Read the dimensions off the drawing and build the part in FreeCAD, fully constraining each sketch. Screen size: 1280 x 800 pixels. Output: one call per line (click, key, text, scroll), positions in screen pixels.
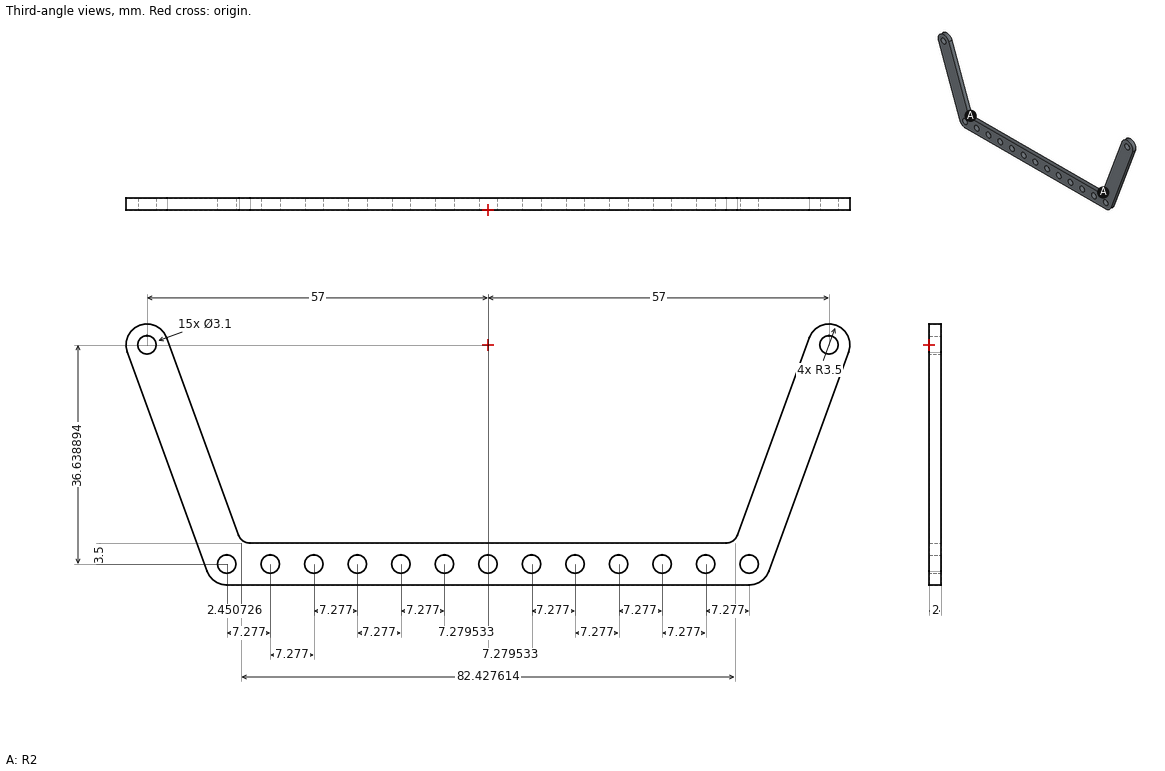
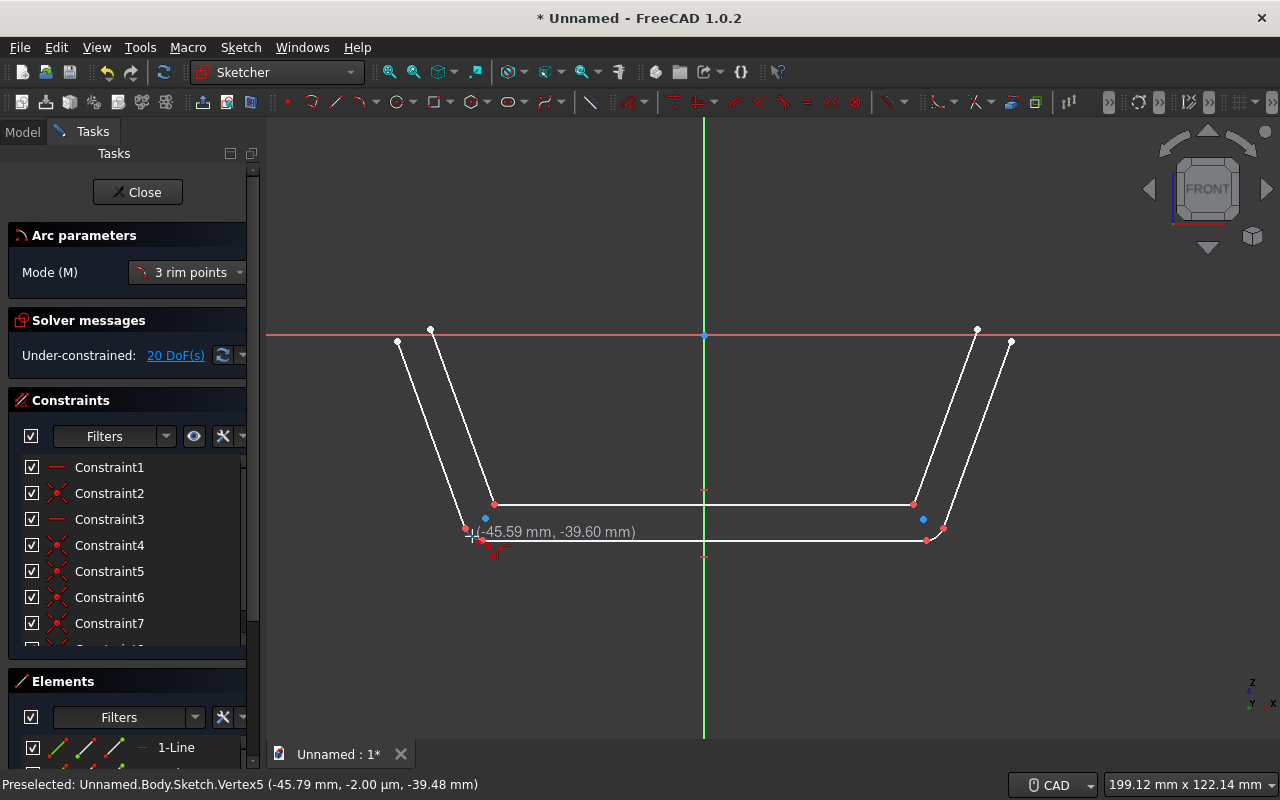
scroll(397, 341, up, 5)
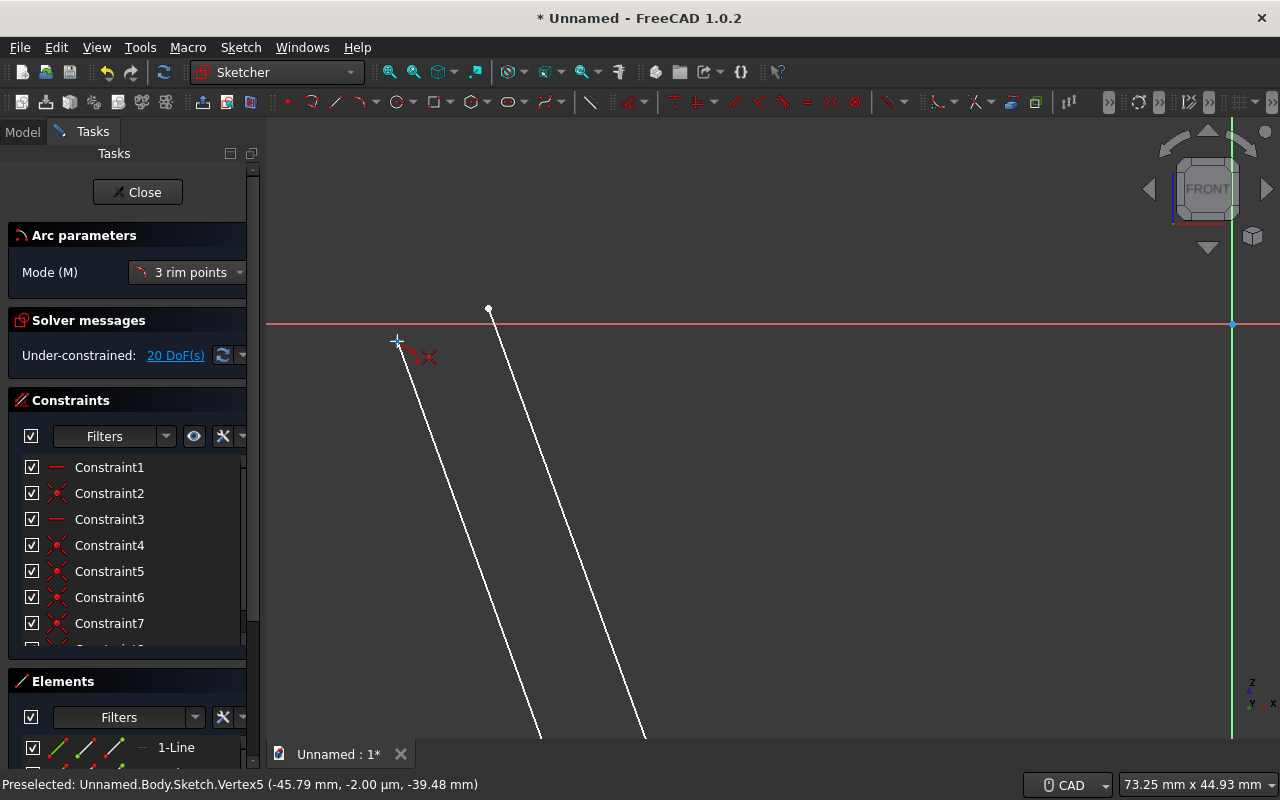
click(398, 341)
click(489, 308)
click(427, 279)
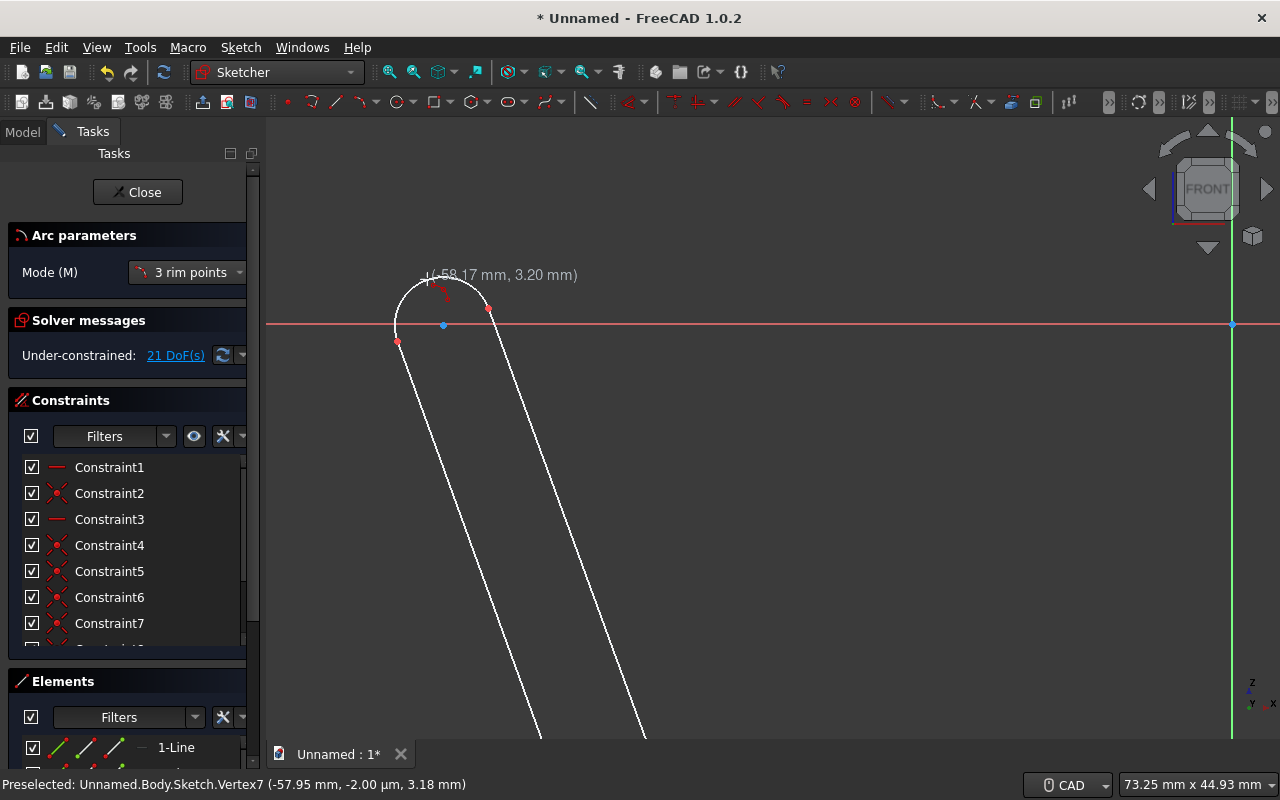
scroll(397, 340, down, 5)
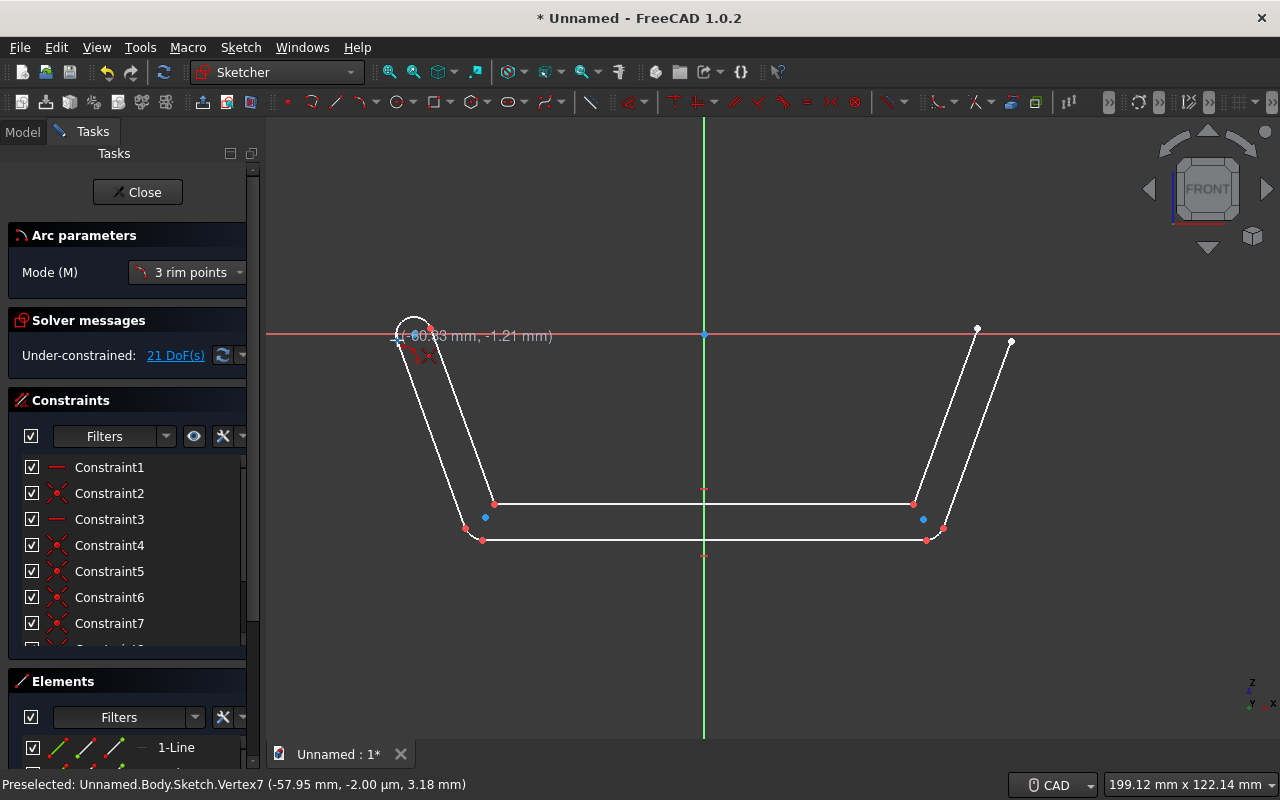
scroll(978, 328, up, 5)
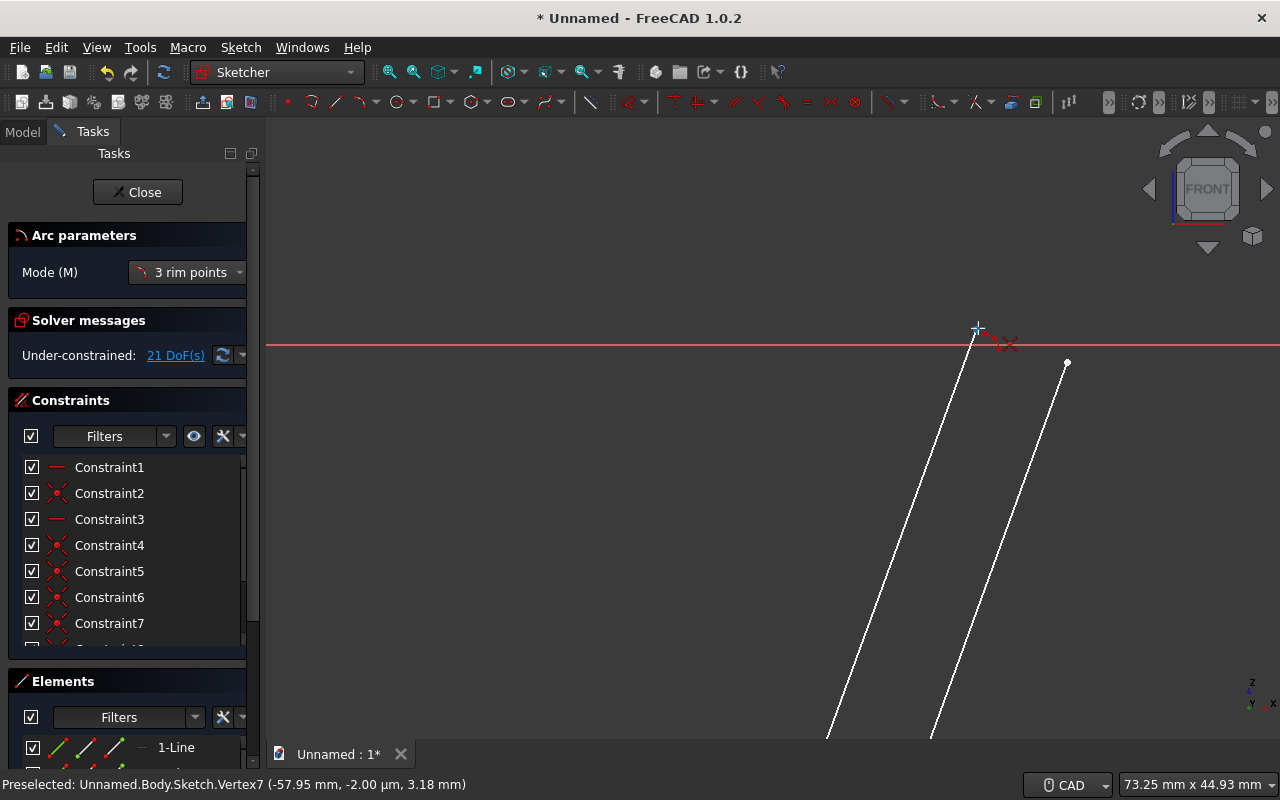
click(977, 329)
click(1067, 363)
click(1039, 299)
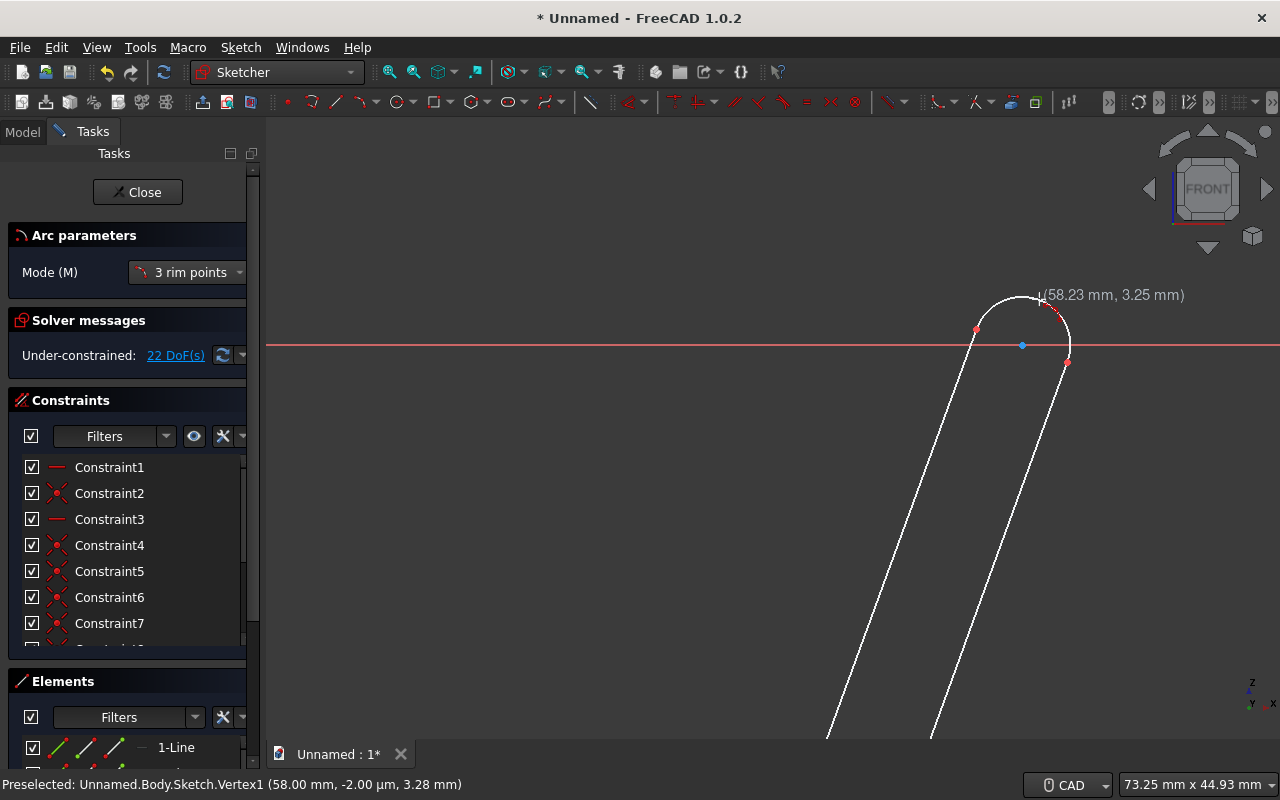
key(g)
key(c)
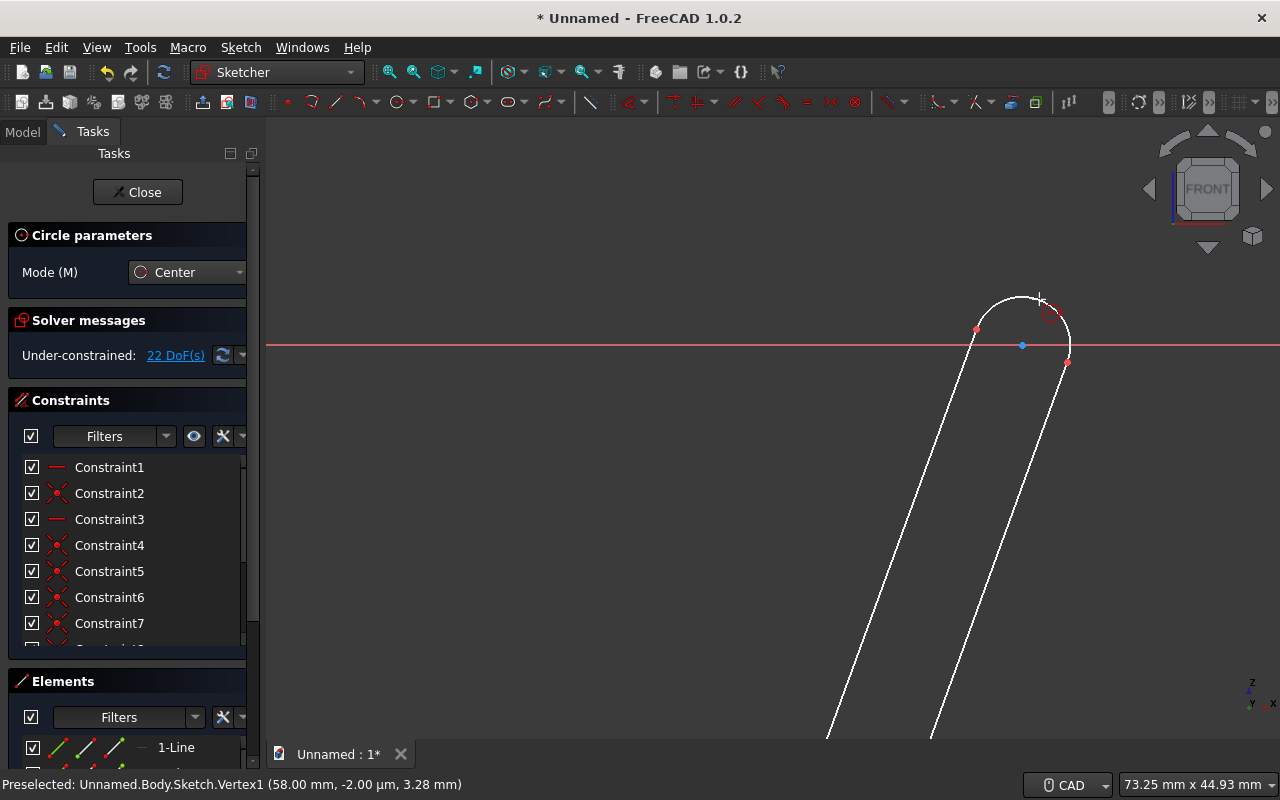
scroll(979, 328, down, 5)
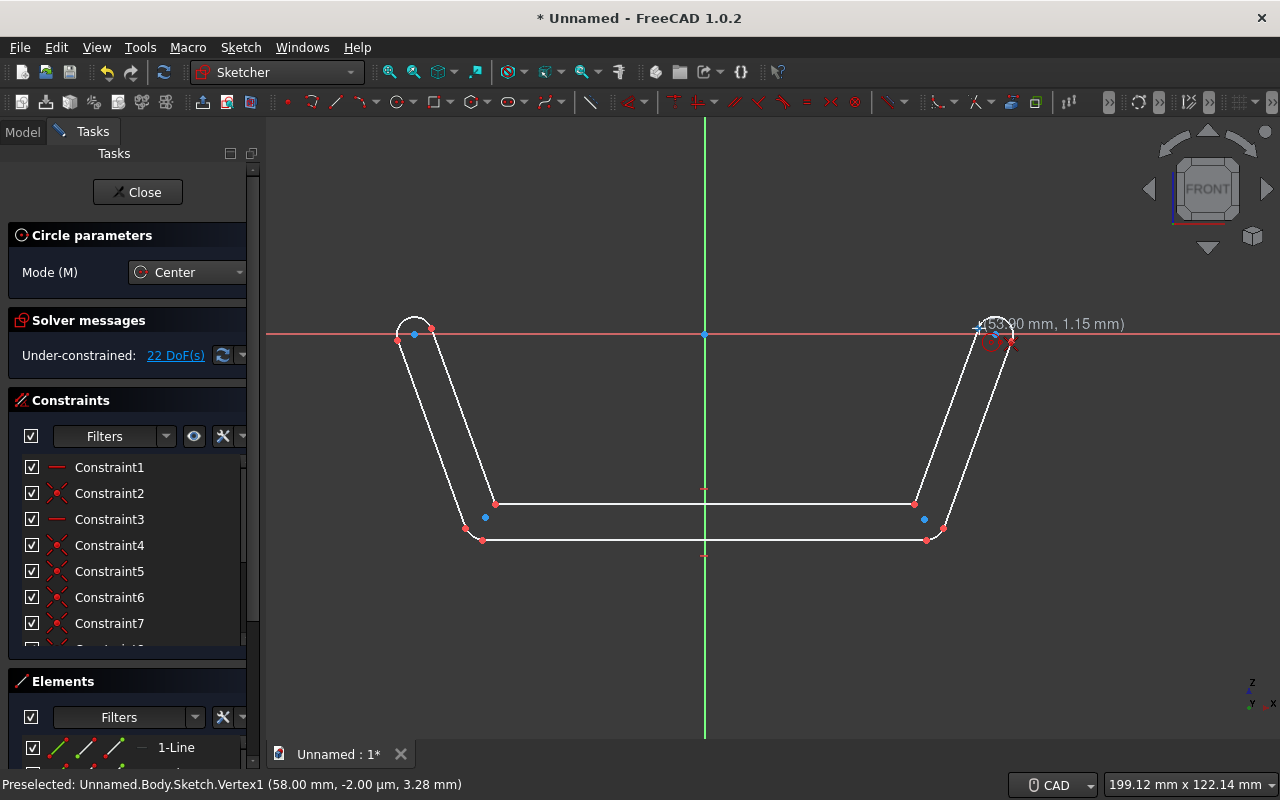
scroll(415, 334, up, 6)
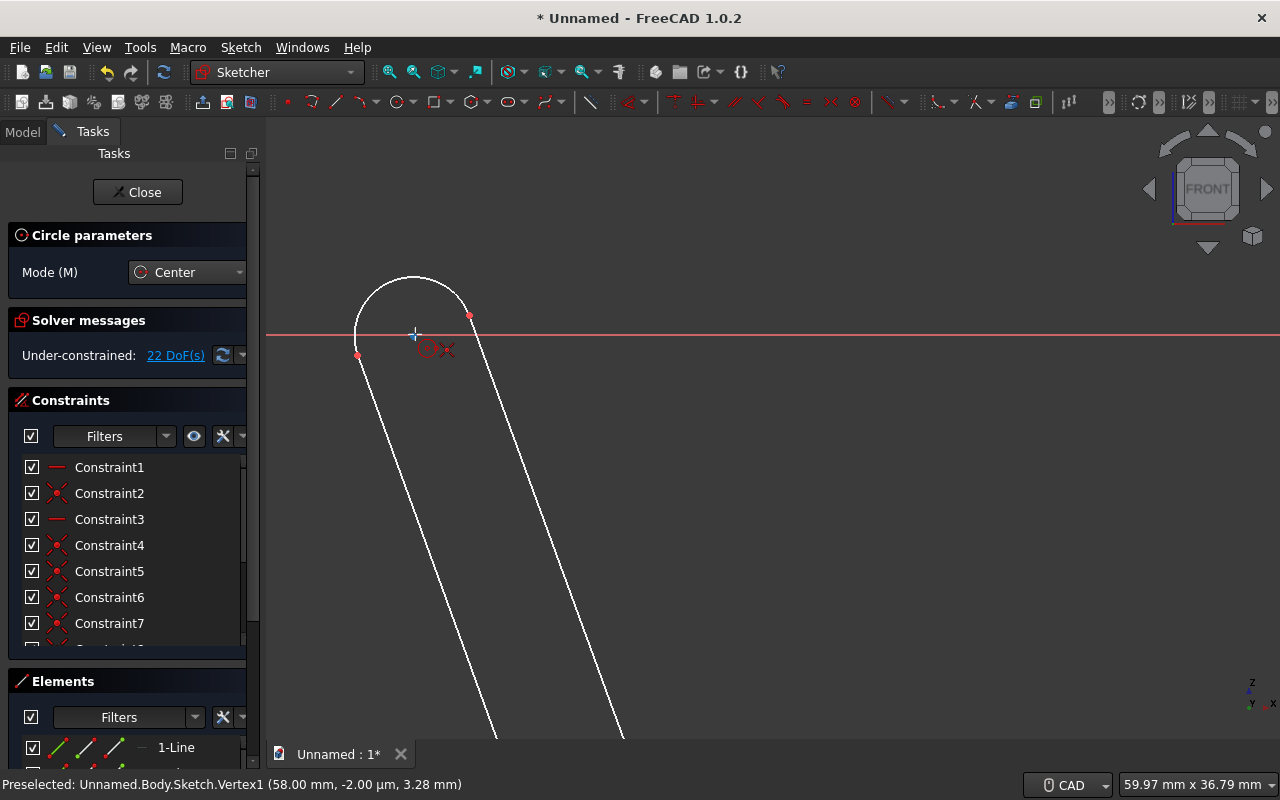
click(414, 335)
move(432, 316)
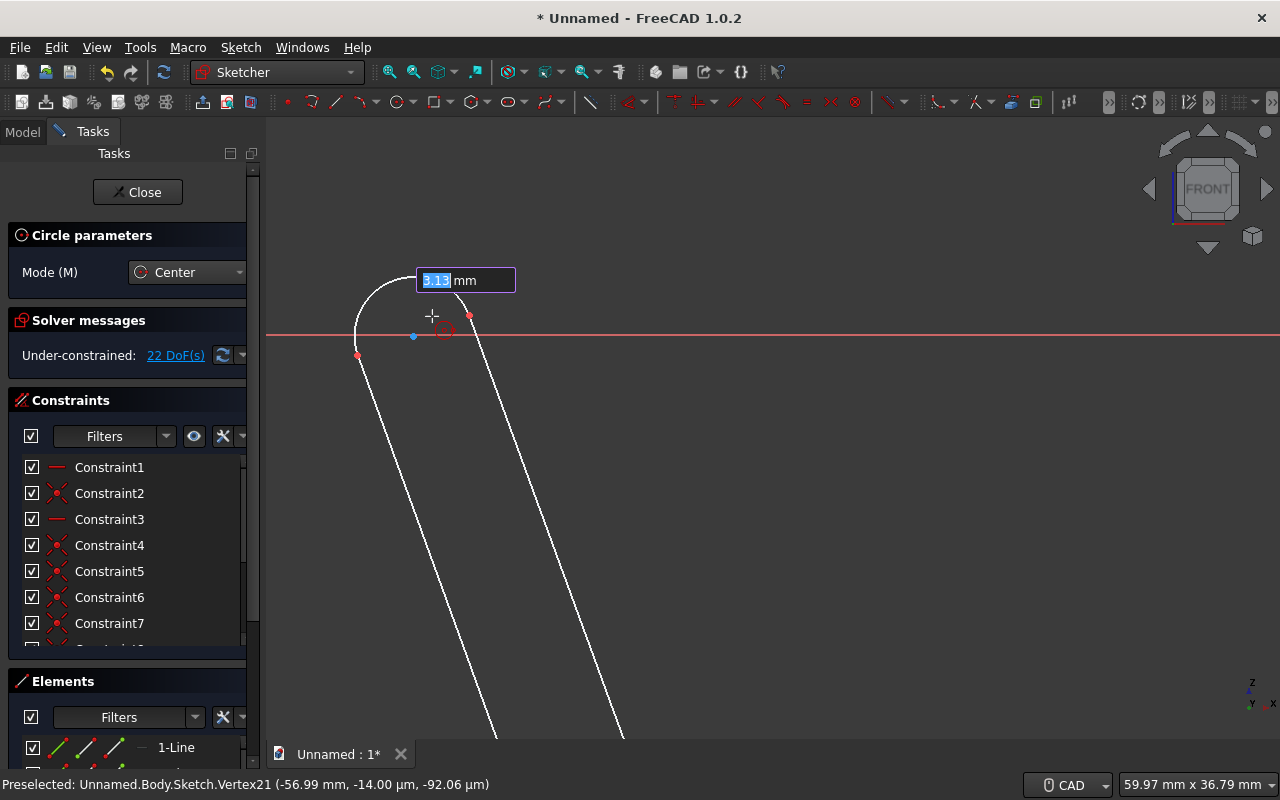
text(3.1)
key(Return)